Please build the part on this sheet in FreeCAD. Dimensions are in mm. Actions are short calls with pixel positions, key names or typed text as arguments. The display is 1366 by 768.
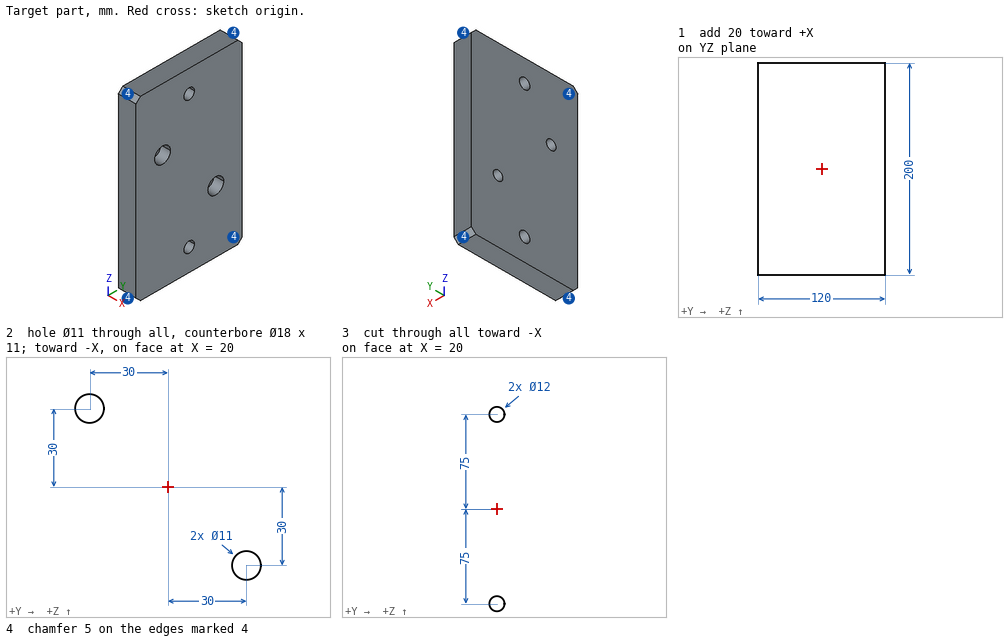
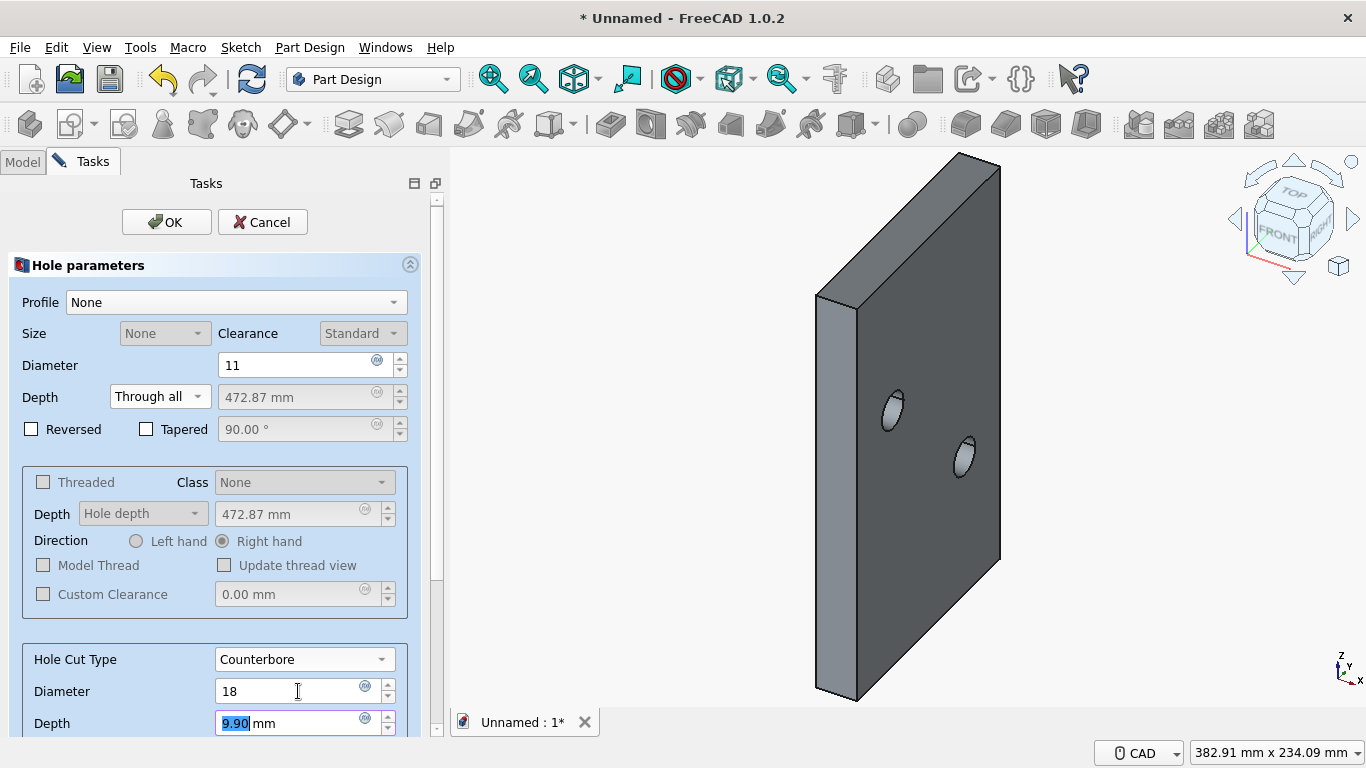
text(11)
key(Tab)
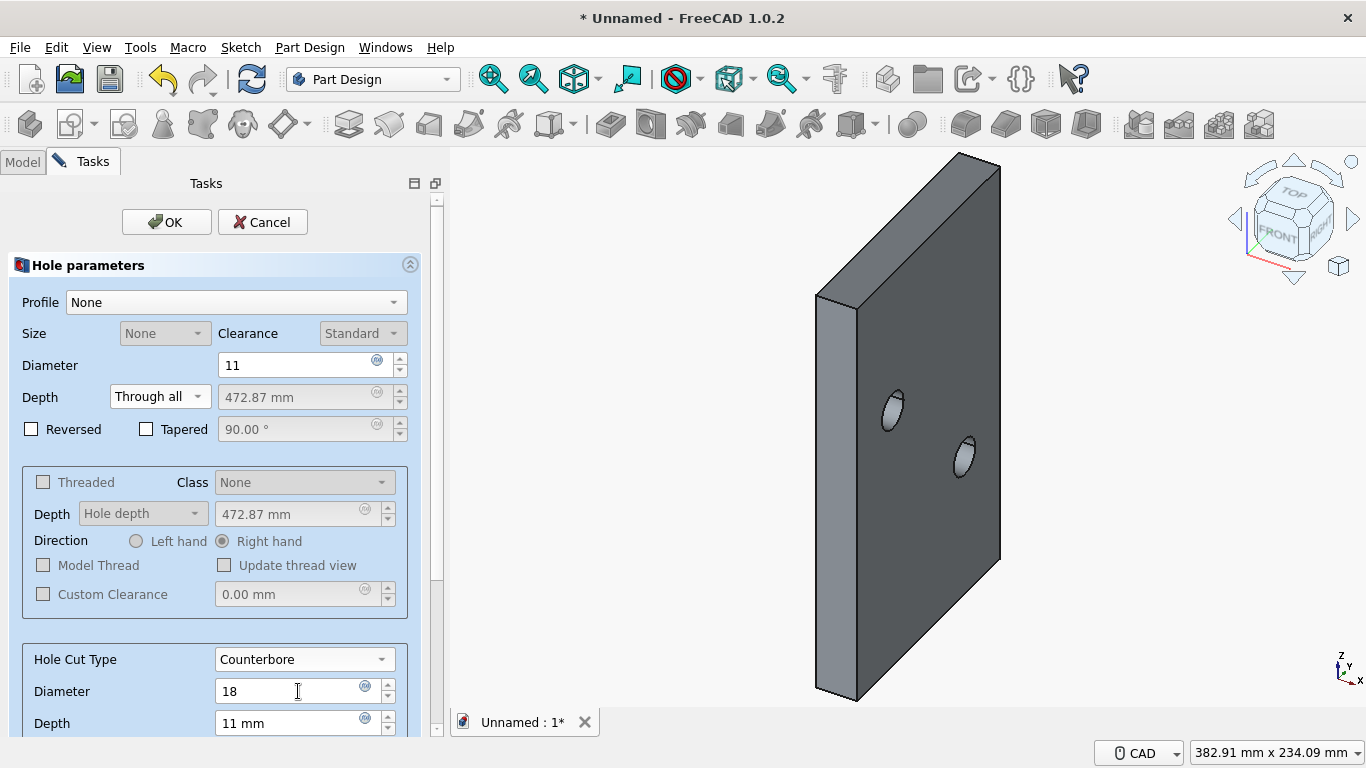
click(167, 222)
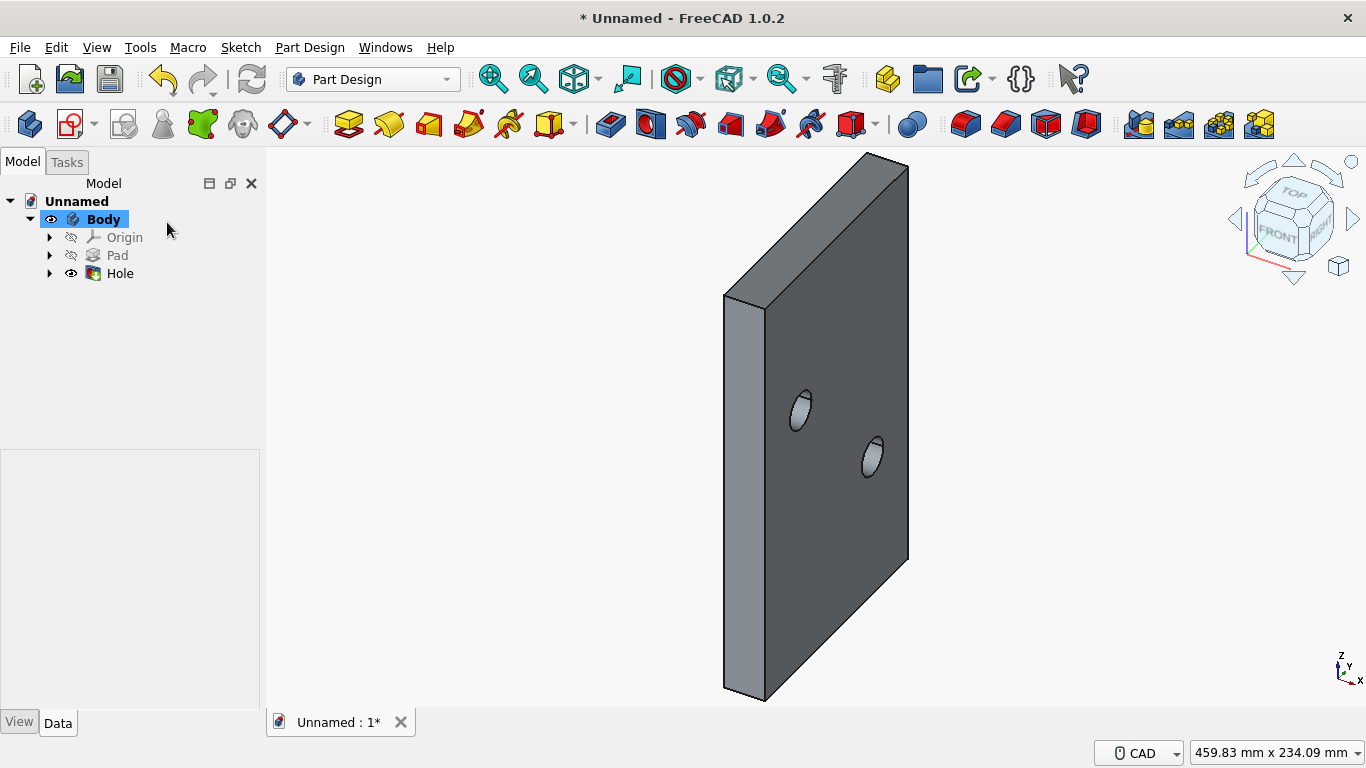
click(816, 565)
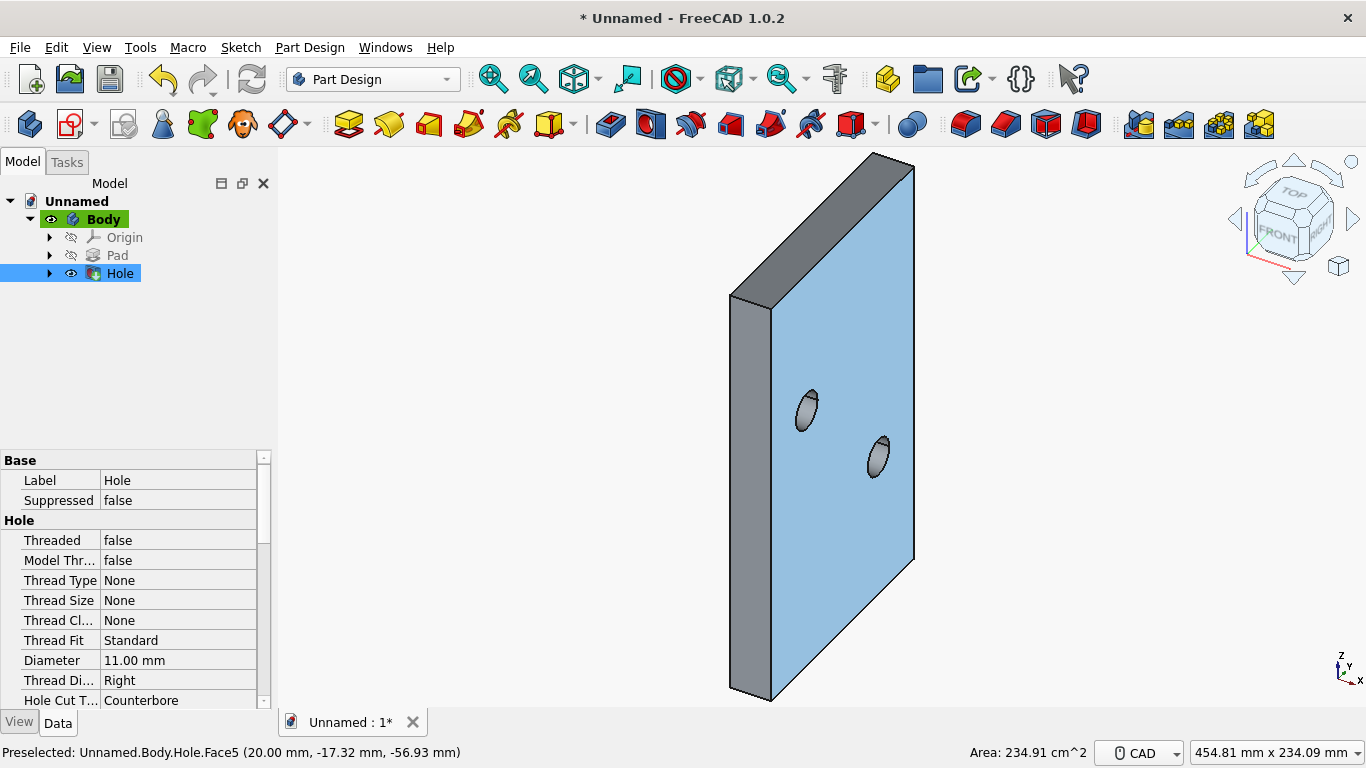
click(70, 124)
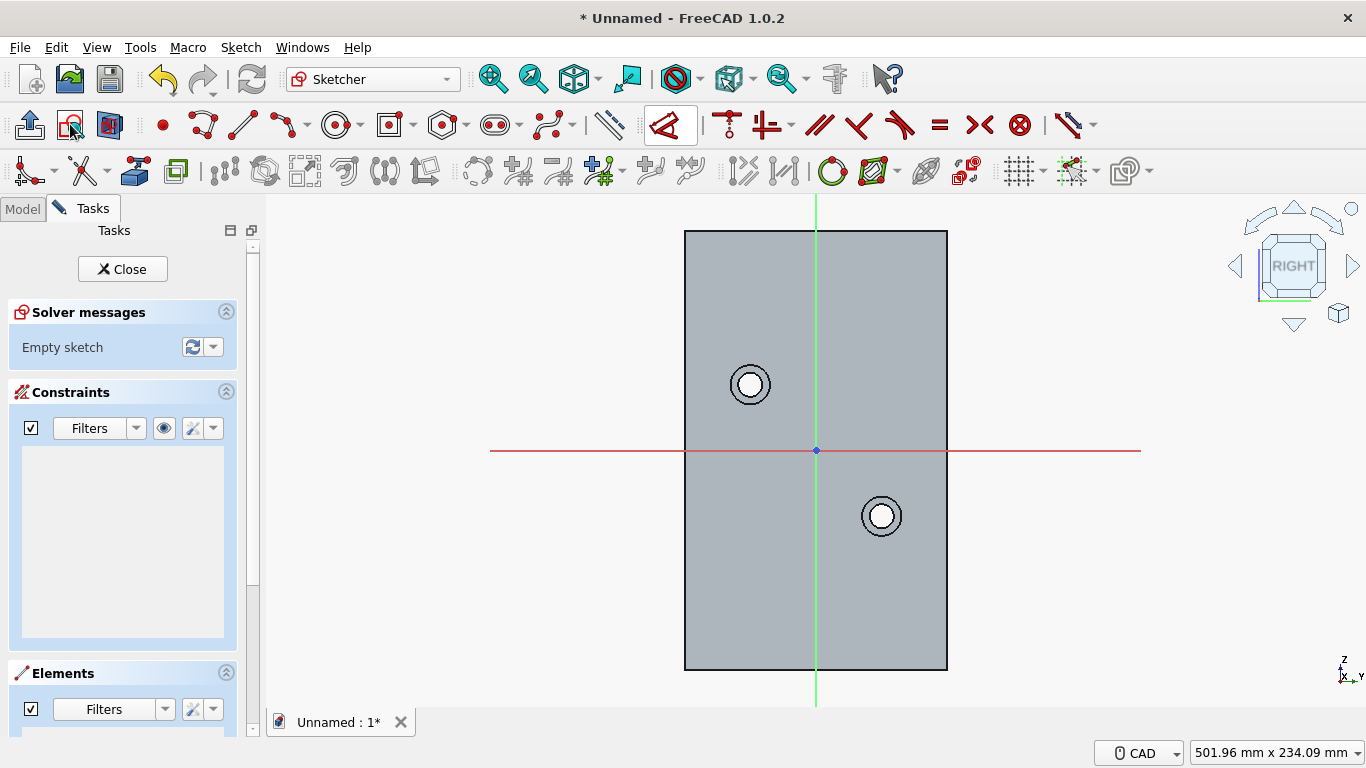
key(g)
key(c)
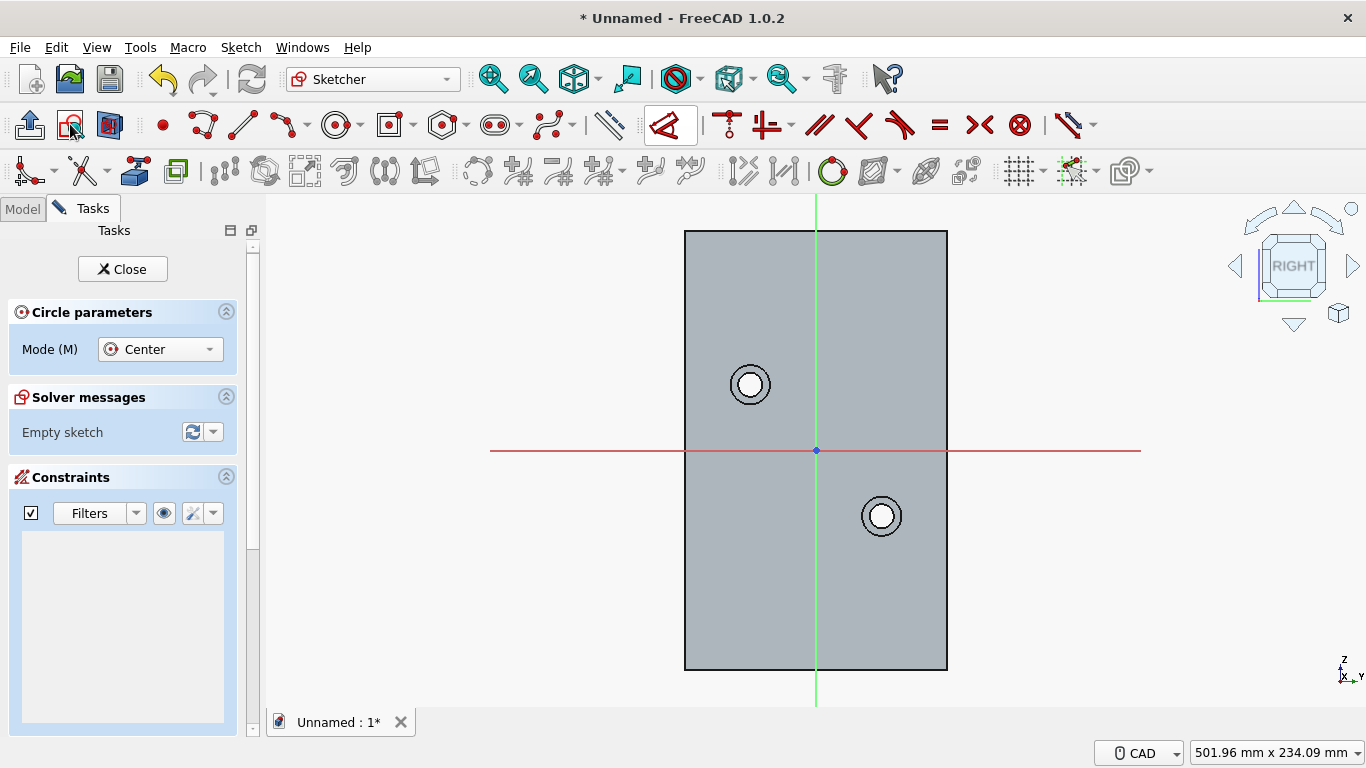
scroll(816, 286, up, 3)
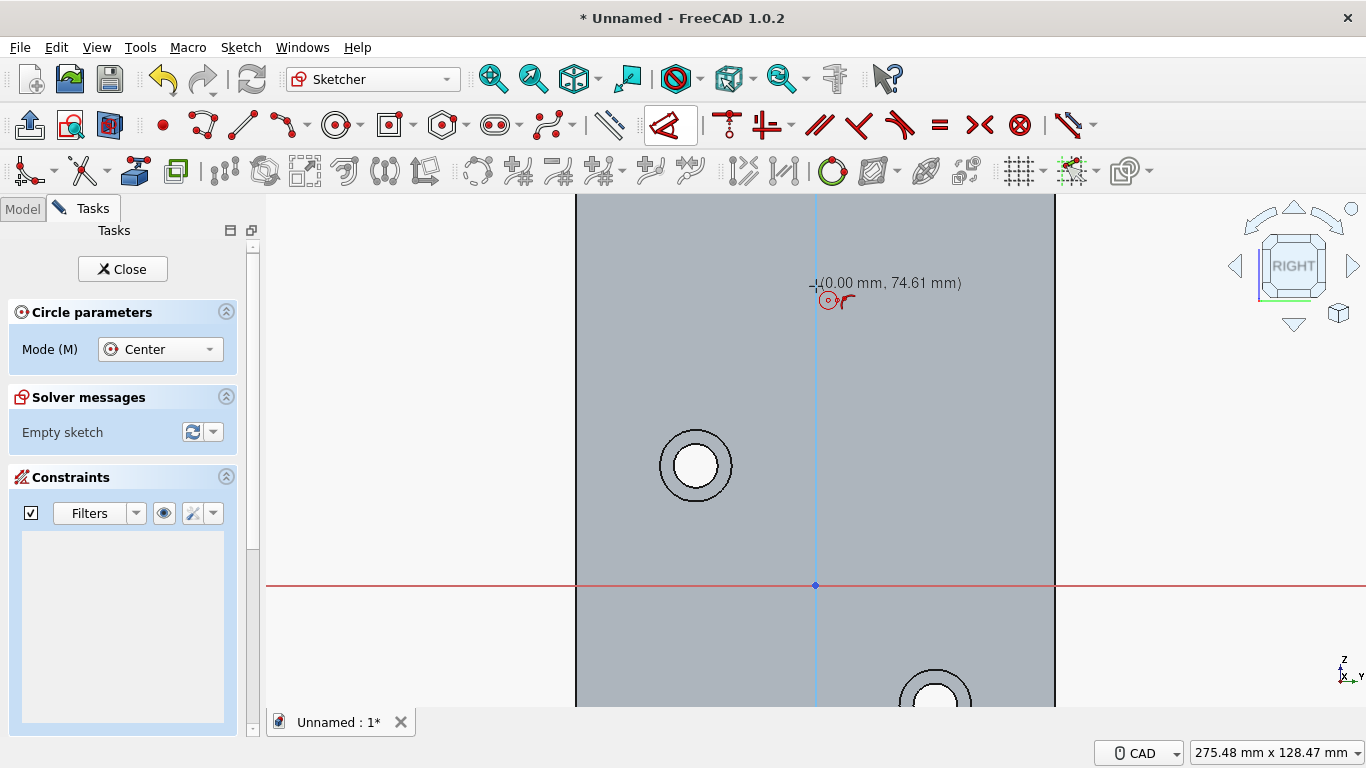
click(816, 286)
move(833, 269)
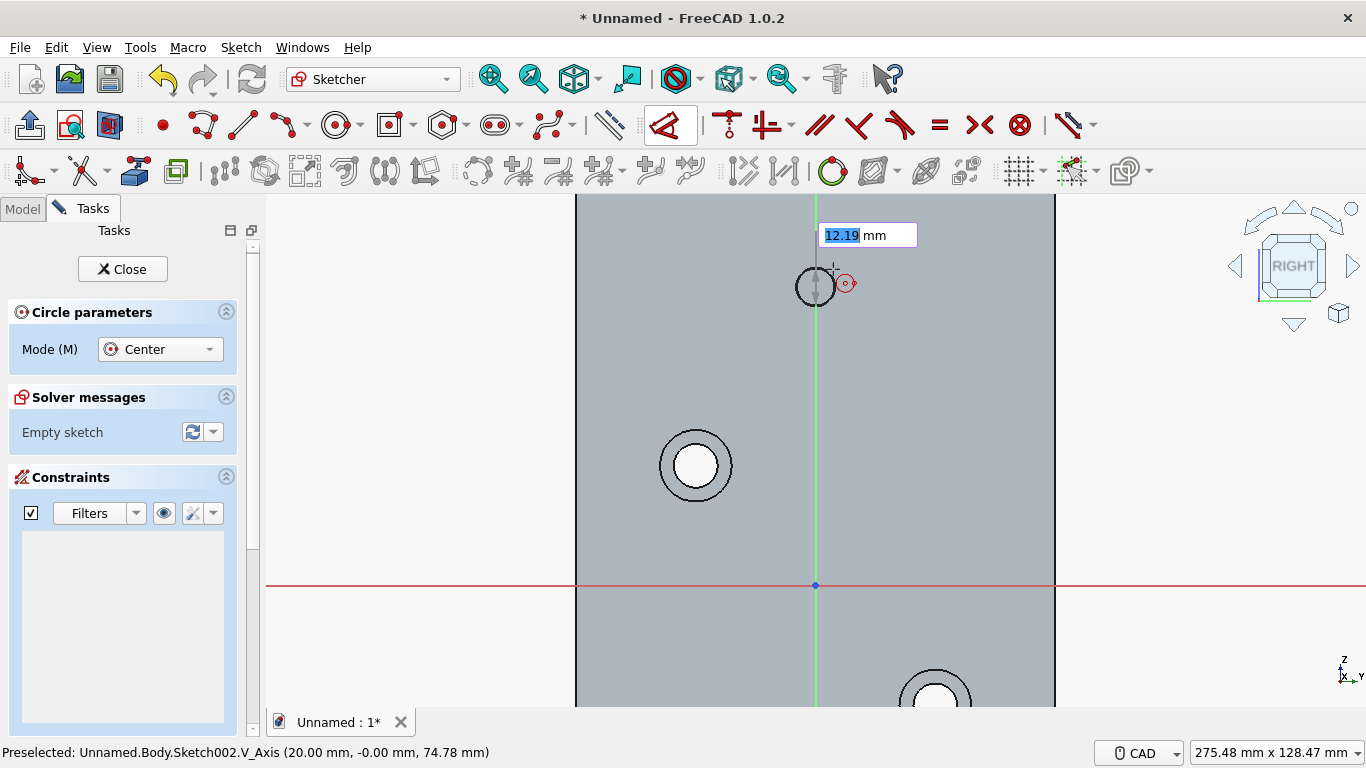
text(12)
key(Return)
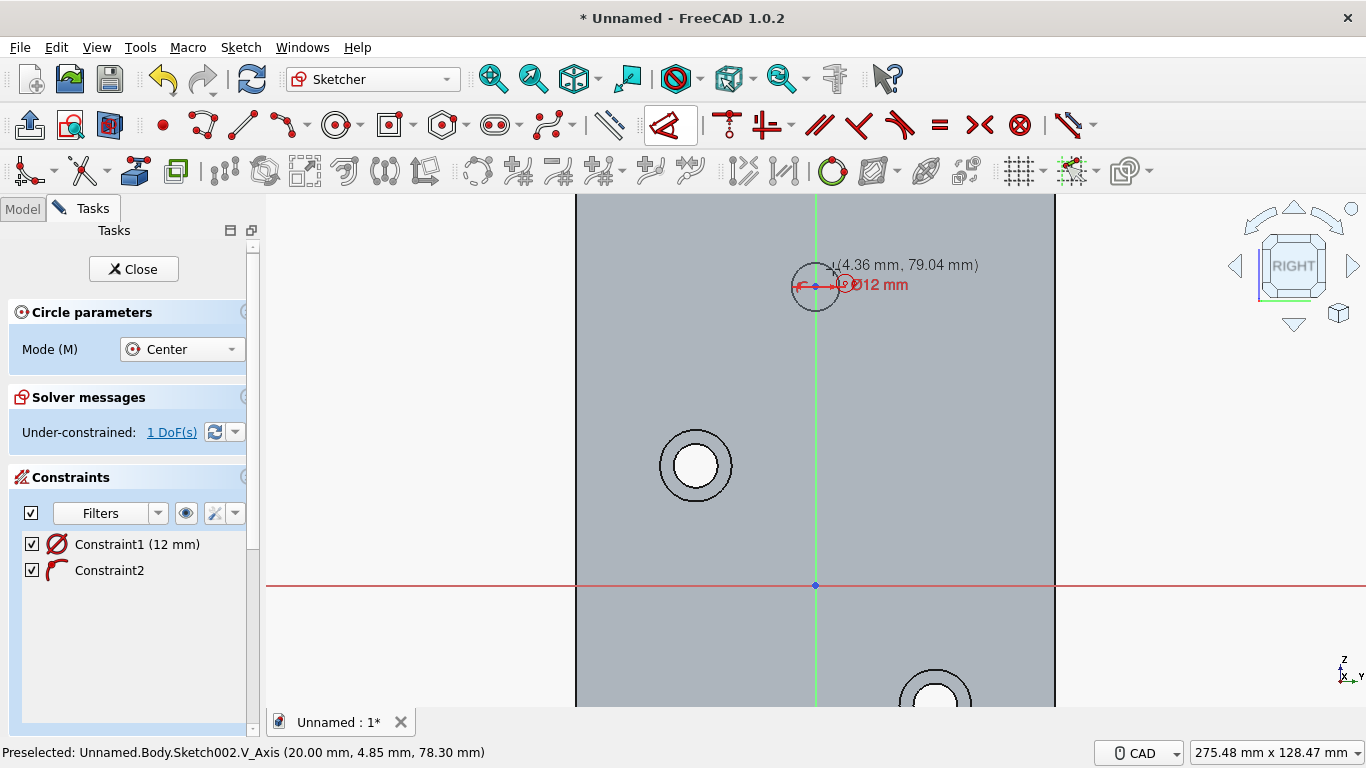
scroll(665, 286, down, 3)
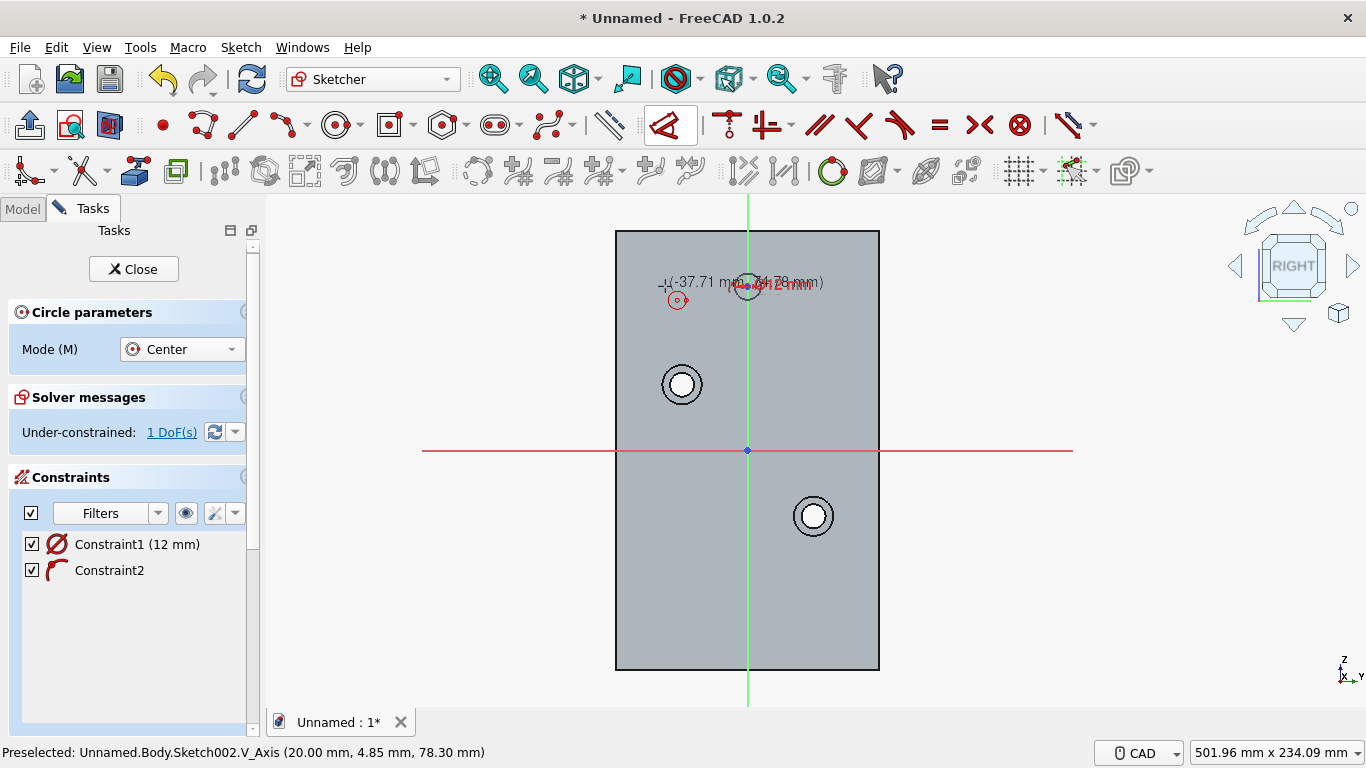
scroll(748, 615, up, 3)